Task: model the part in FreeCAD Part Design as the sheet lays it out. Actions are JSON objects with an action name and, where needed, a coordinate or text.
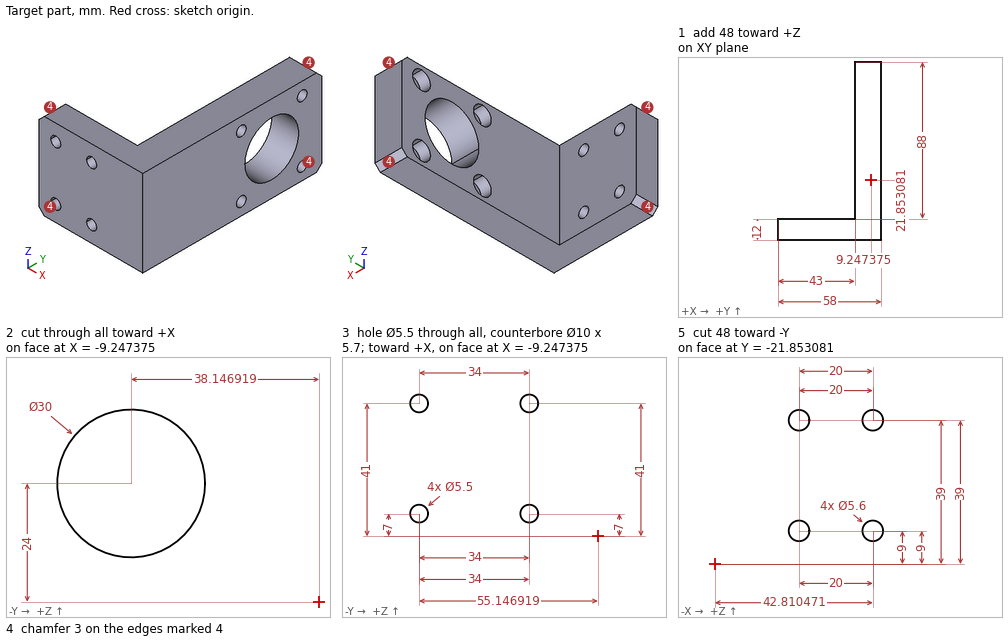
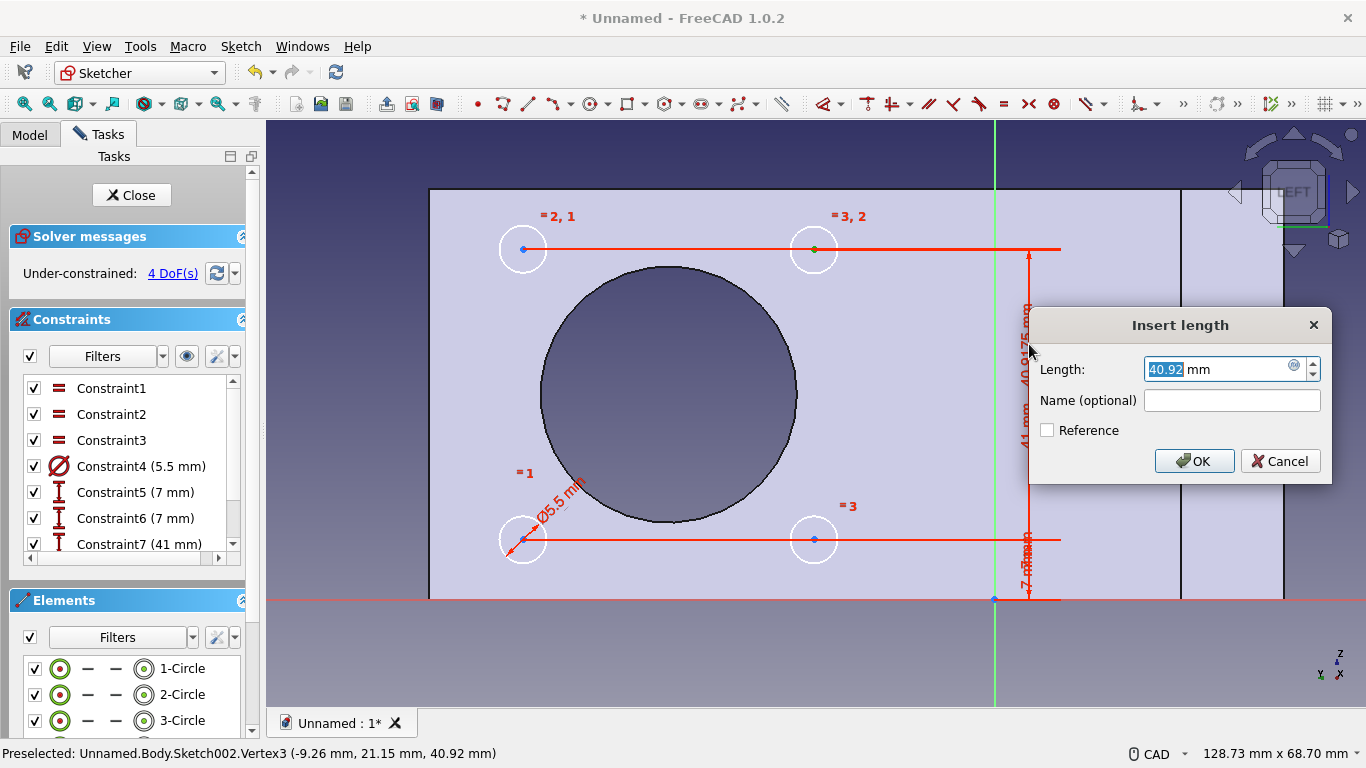
{"action": "type", "text": "41"}
{"action": "key", "text": "Return"}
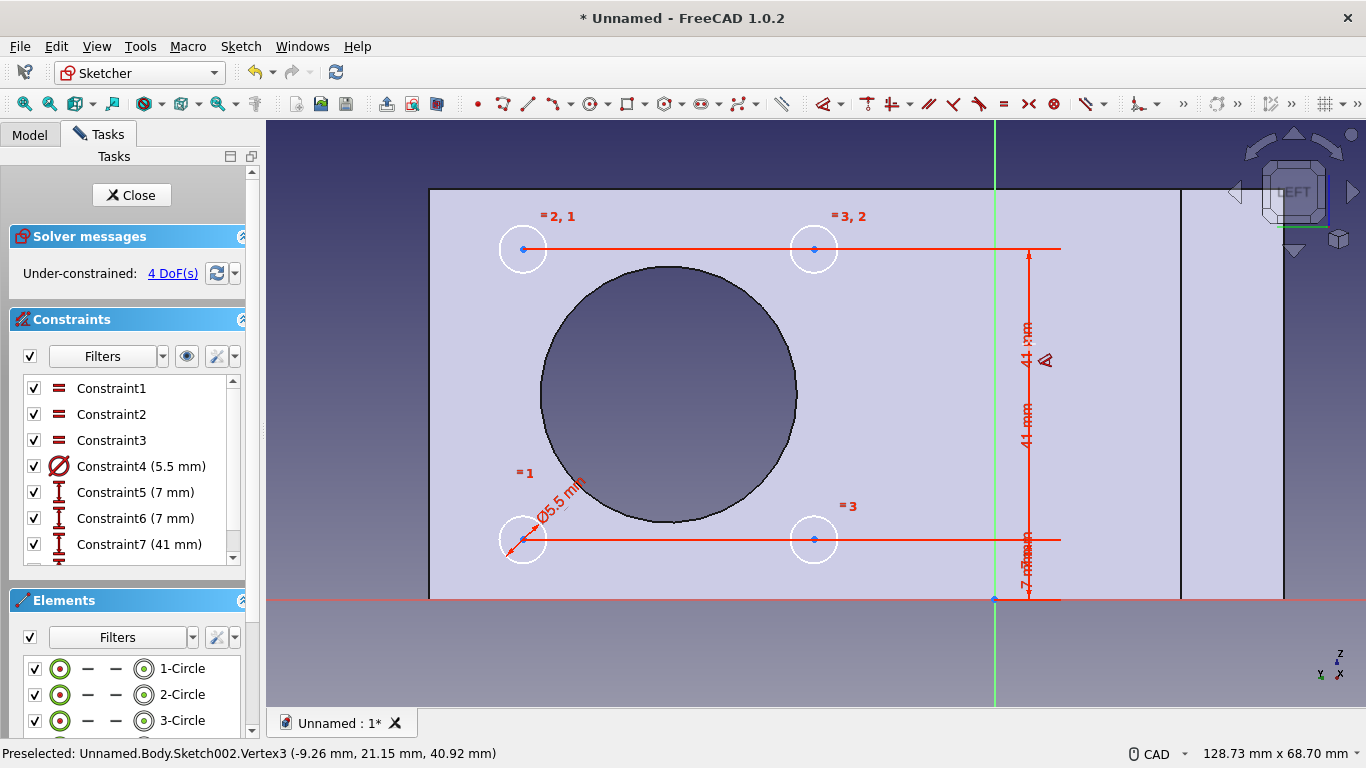
{"action": "left_click", "coordinate": [523, 249]}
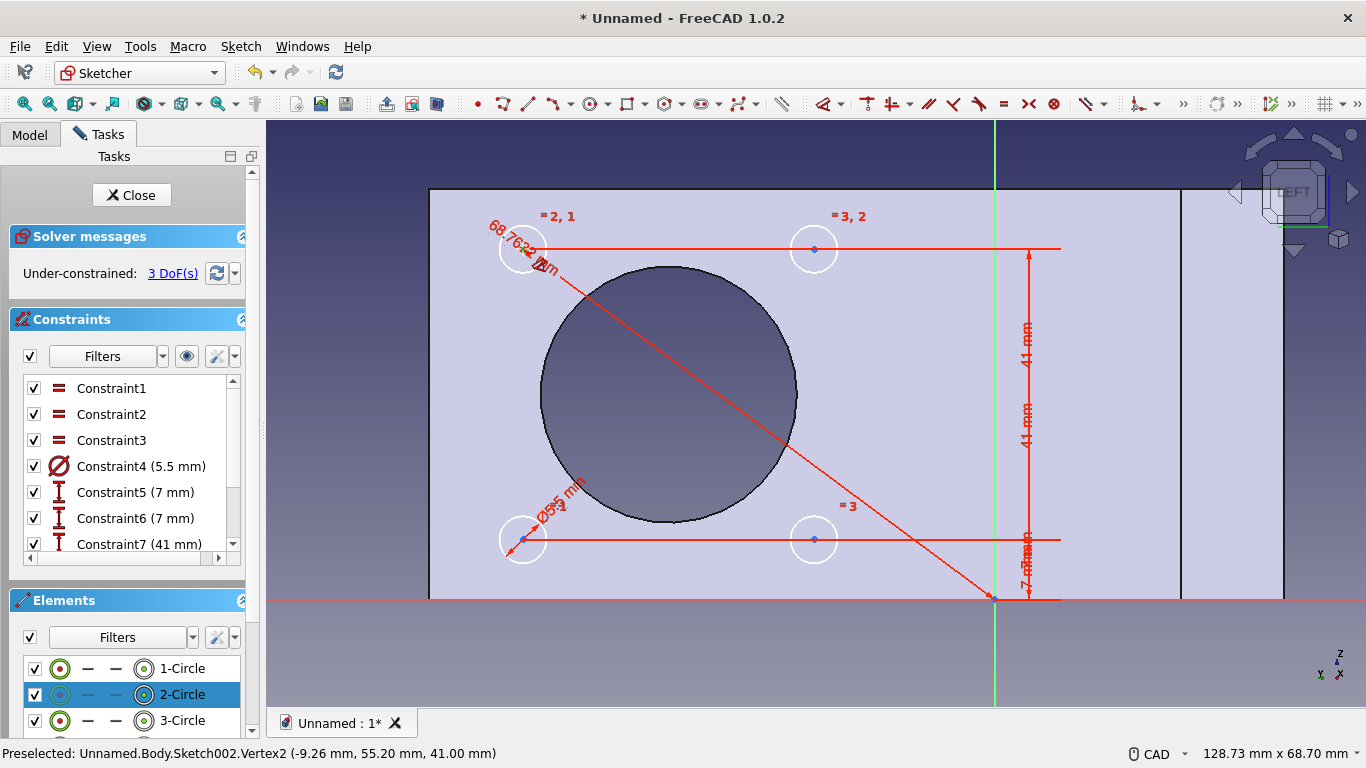
{"action": "left_click", "coordinate": [814, 249]}
{"action": "left_click", "coordinate": [669, 215]}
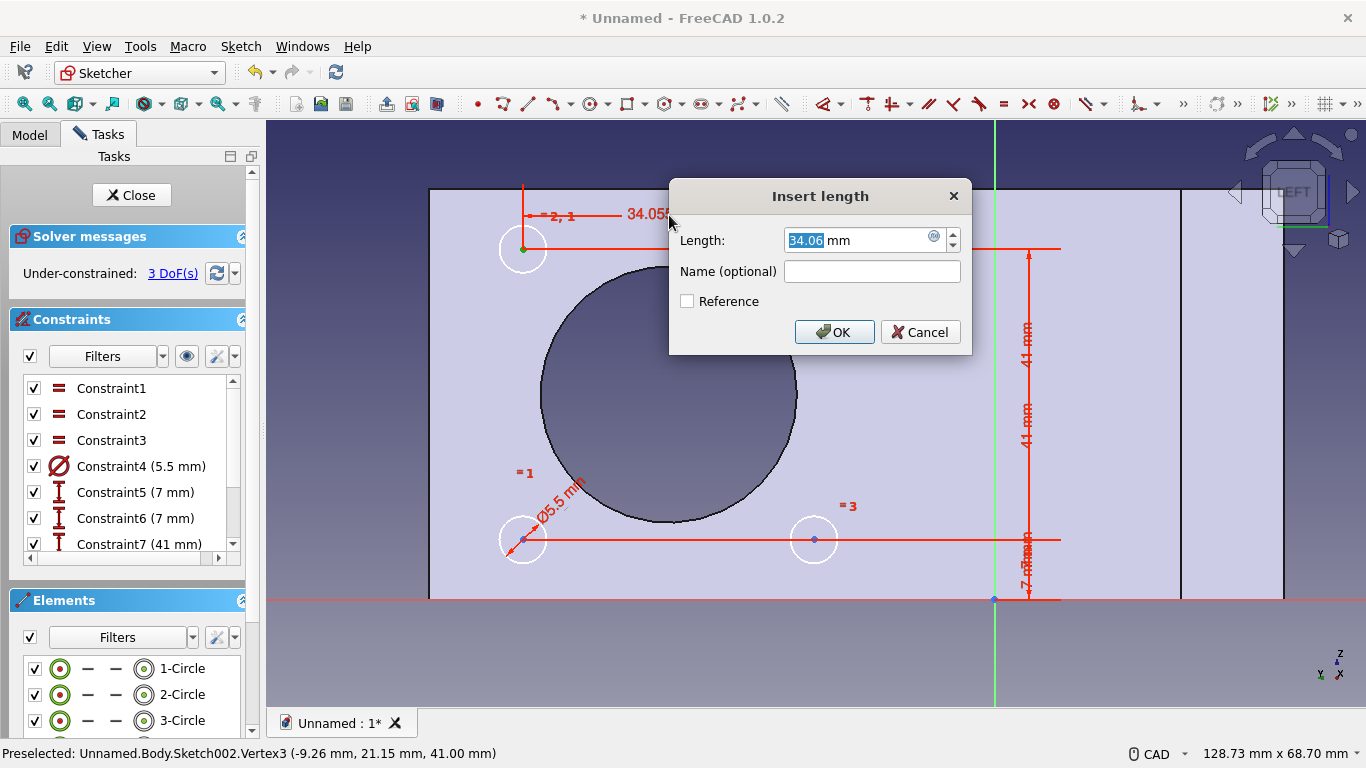
{"action": "type", "text": "34"}
{"action": "key", "text": "Return"}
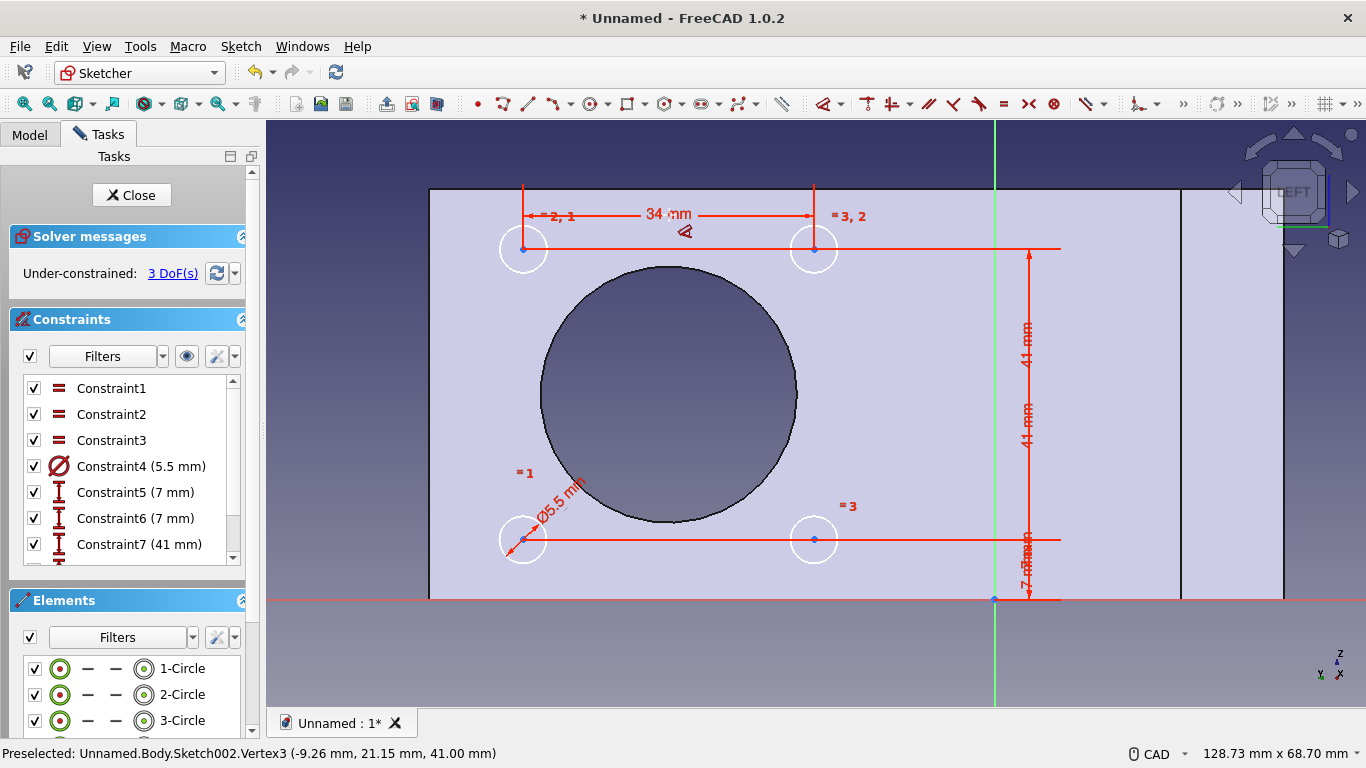
{"action": "left_click", "coordinate": [523, 540]}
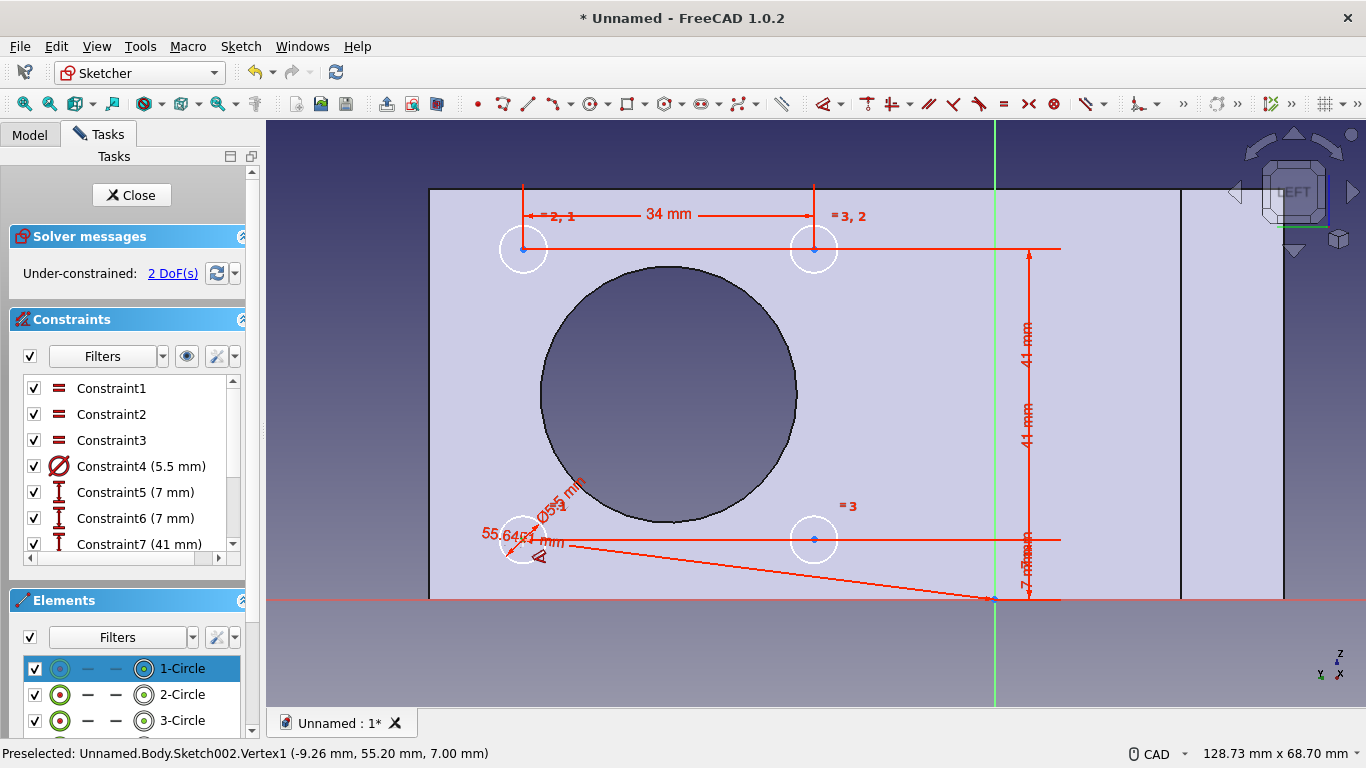
{"action": "left_click", "coordinate": [814, 249]}
{"action": "left_click", "coordinate": [567, 215]}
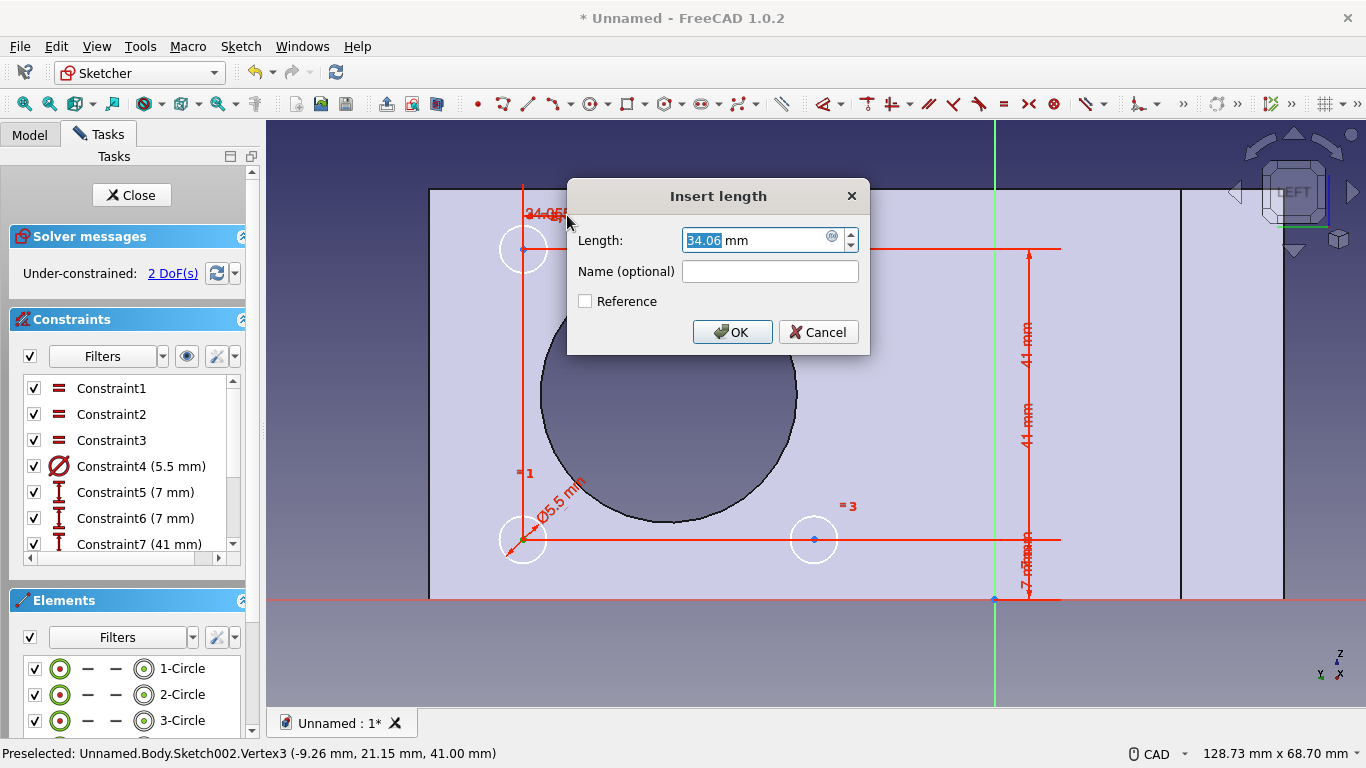
{"action": "type", "text": "34"}
{"action": "key", "text": "Return"}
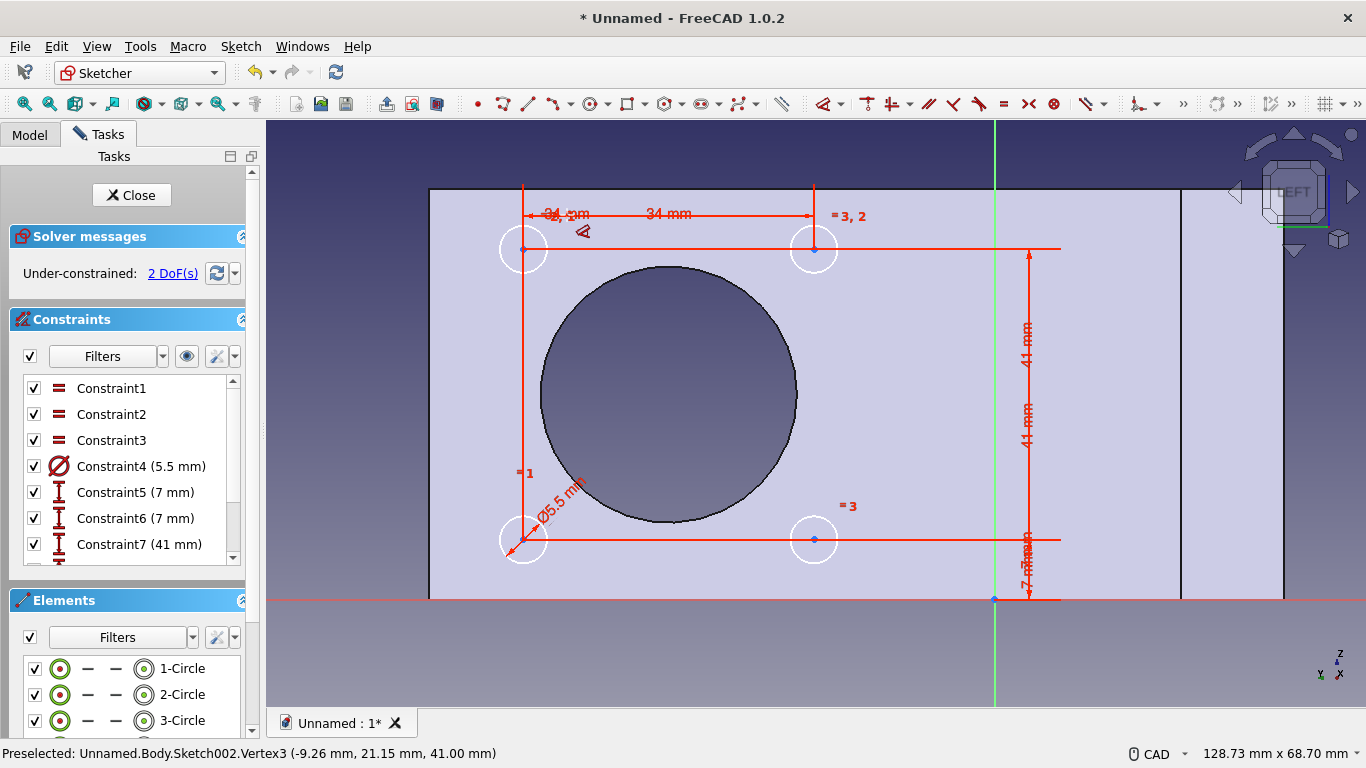
{"action": "left_click", "coordinate": [523, 540]}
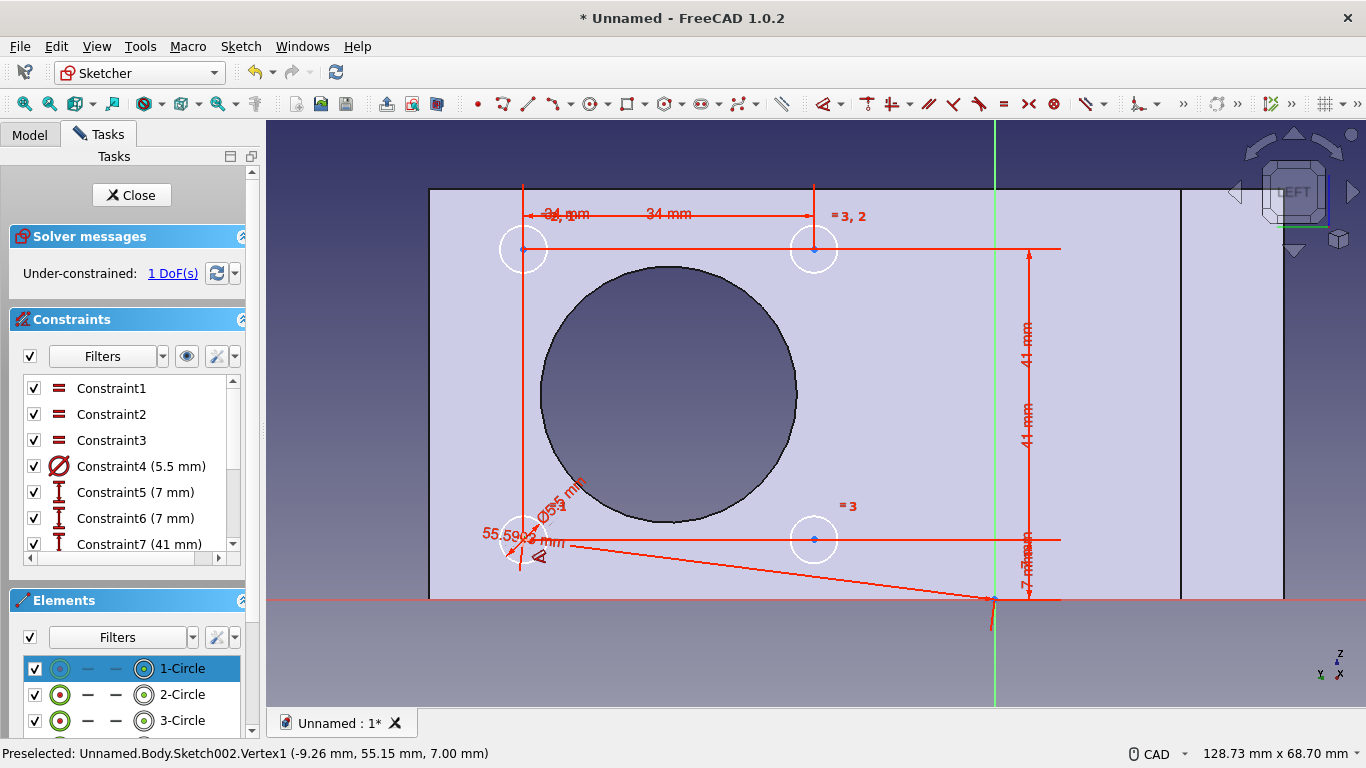
{"action": "left_click", "coordinate": [814, 540]}
{"action": "left_click", "coordinate": [669, 574]}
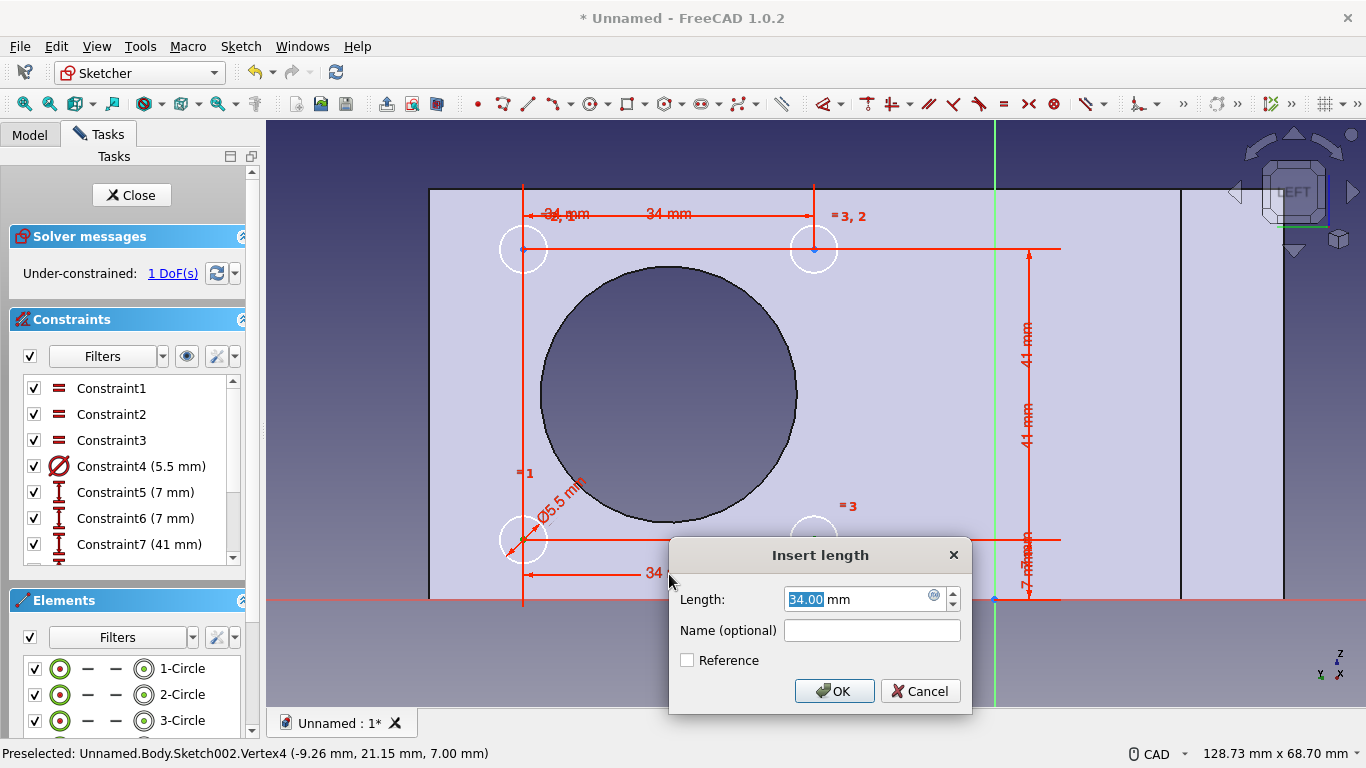
{"action": "type", "text": "34"}
{"action": "key", "text": "Return"}